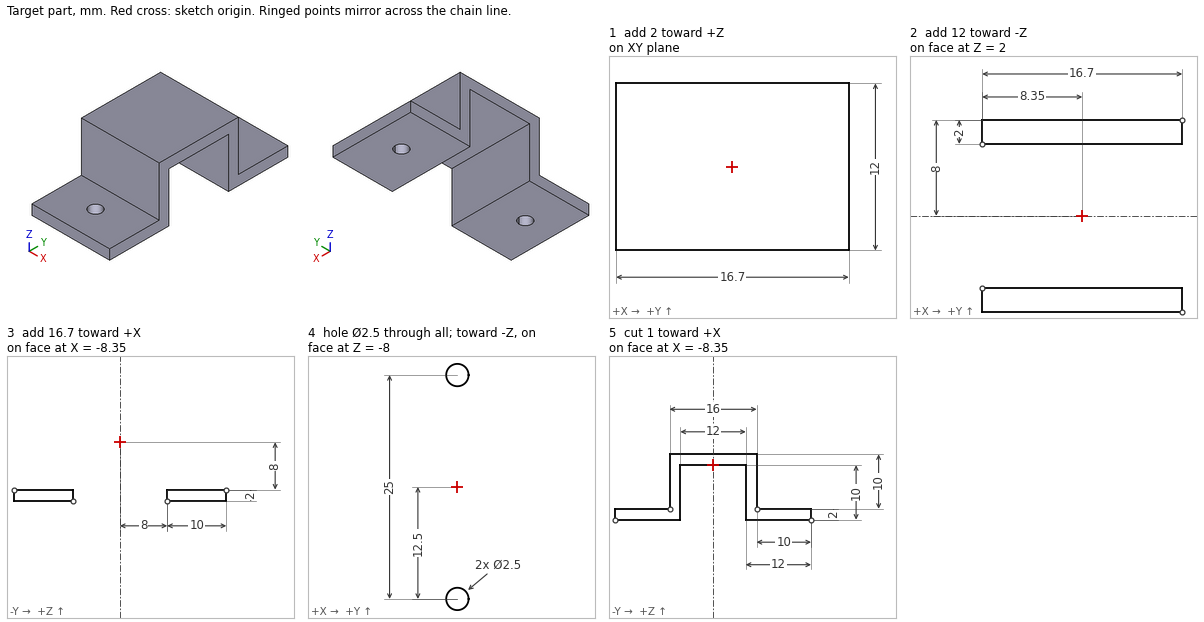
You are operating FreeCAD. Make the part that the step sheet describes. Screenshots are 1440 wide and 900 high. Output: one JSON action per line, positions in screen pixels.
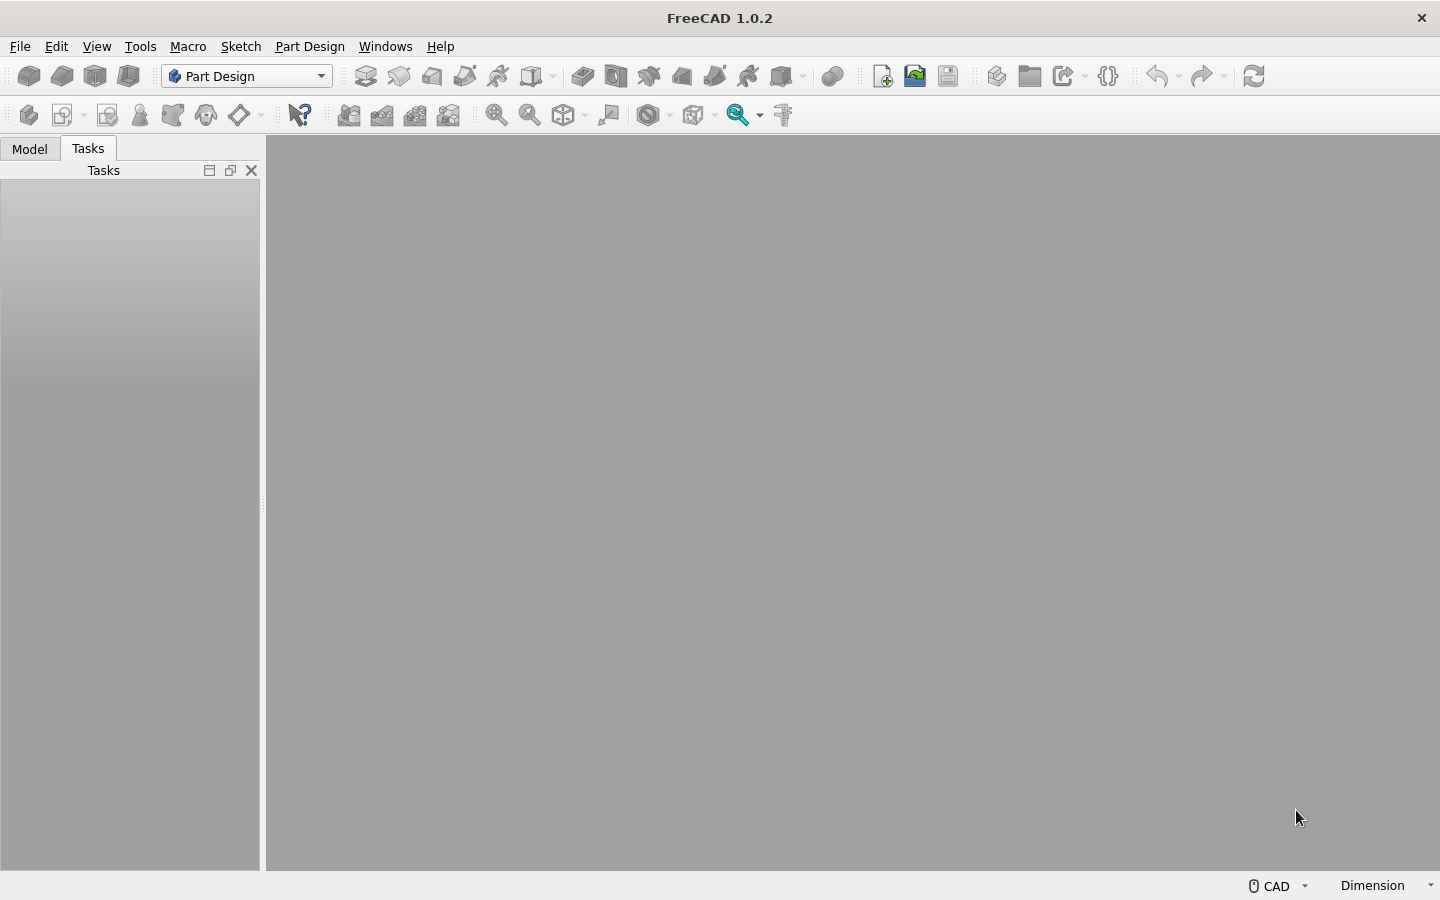
{"action": "left_click", "coordinate": [882, 76]}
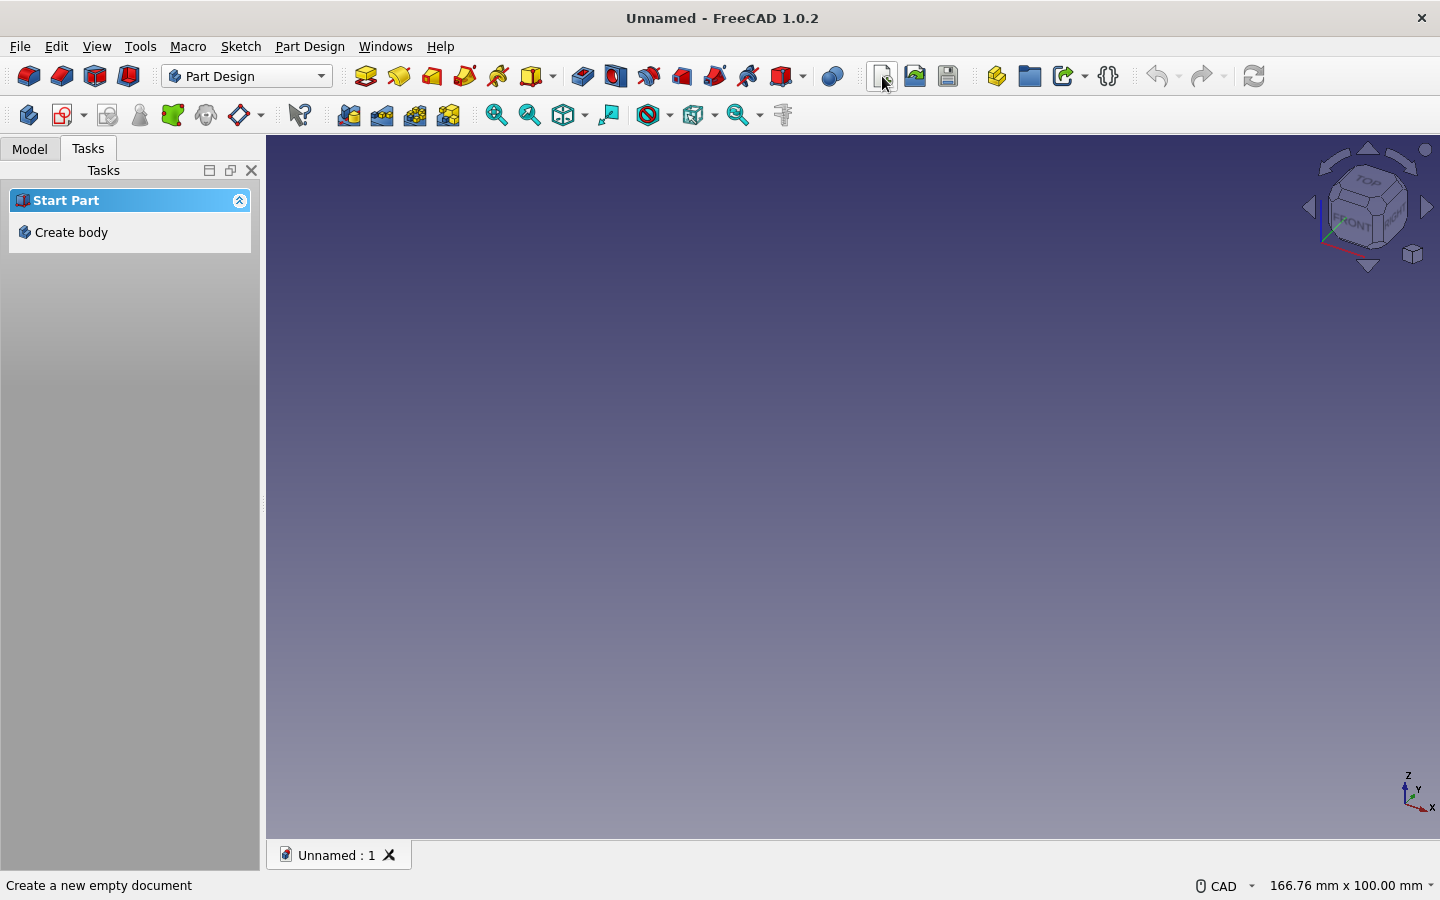
{"action": "left_click", "coordinate": [62, 116]}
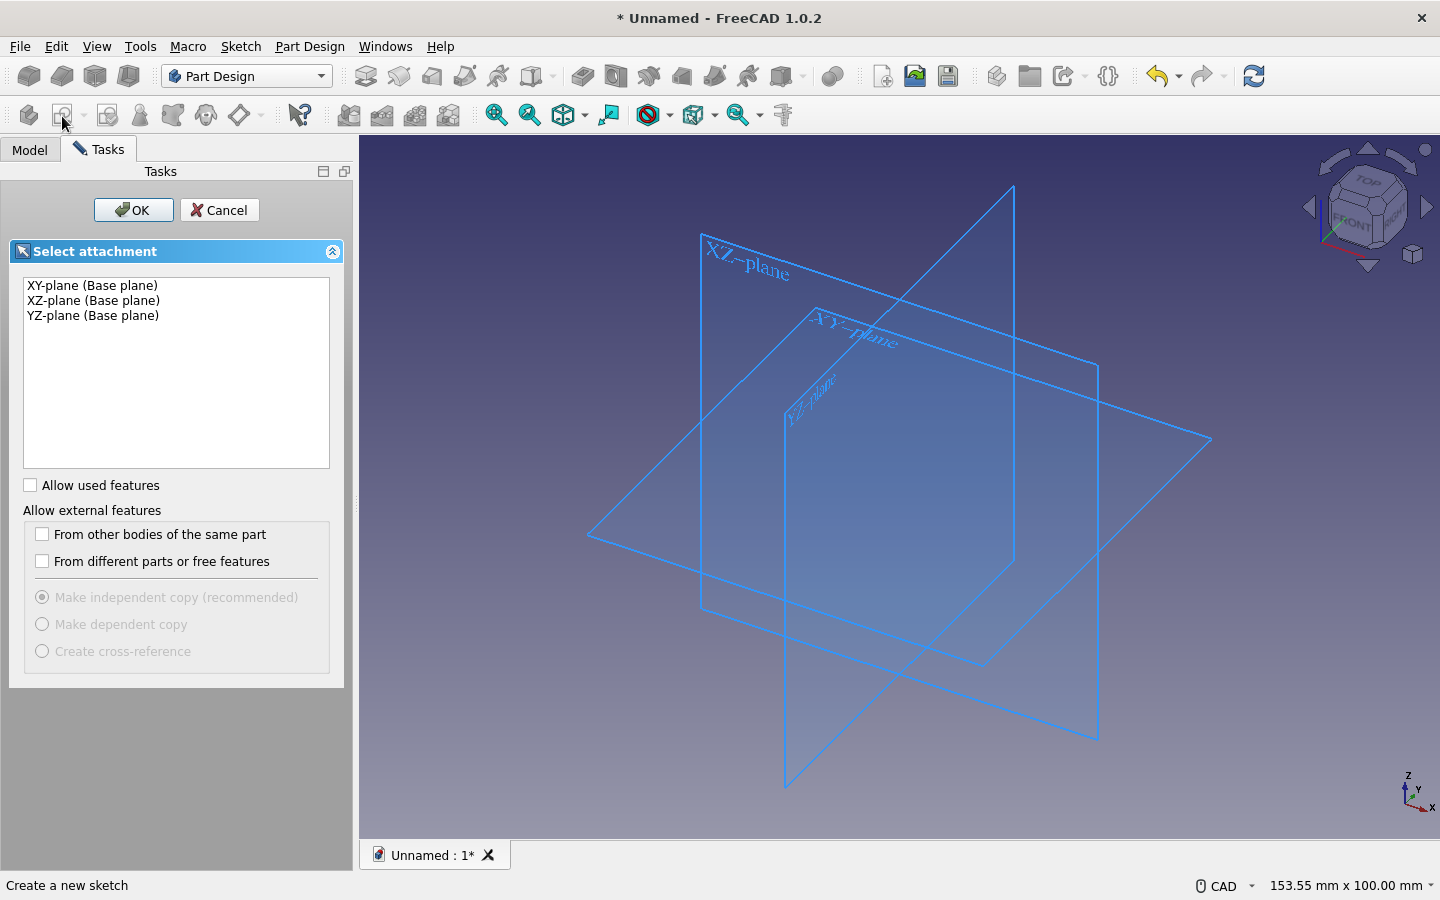
{"action": "left_click", "coordinate": [84, 286]}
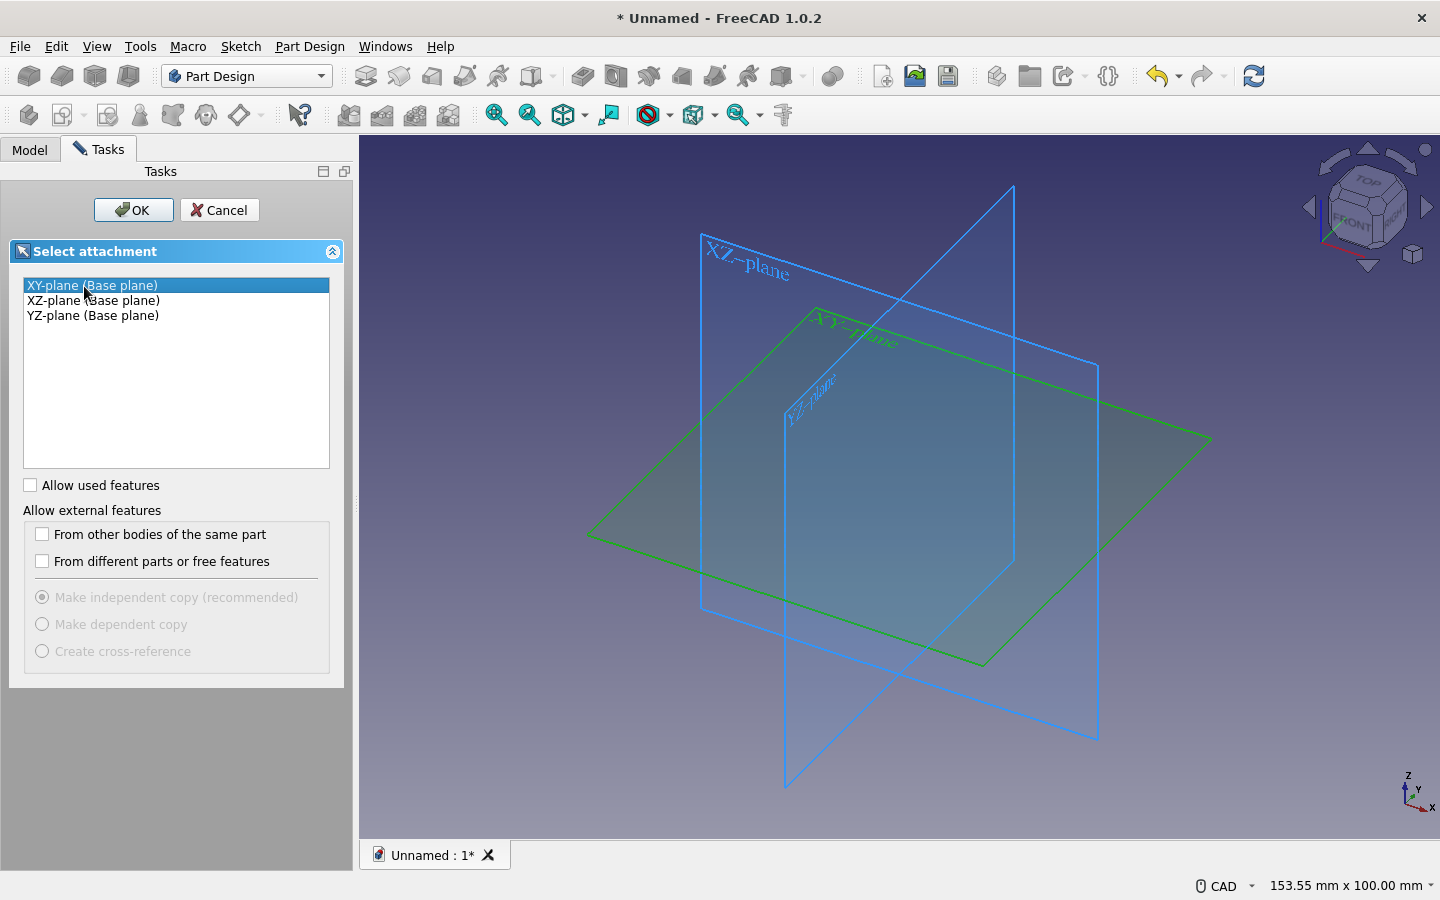
{"action": "left_click", "coordinate": [134, 210]}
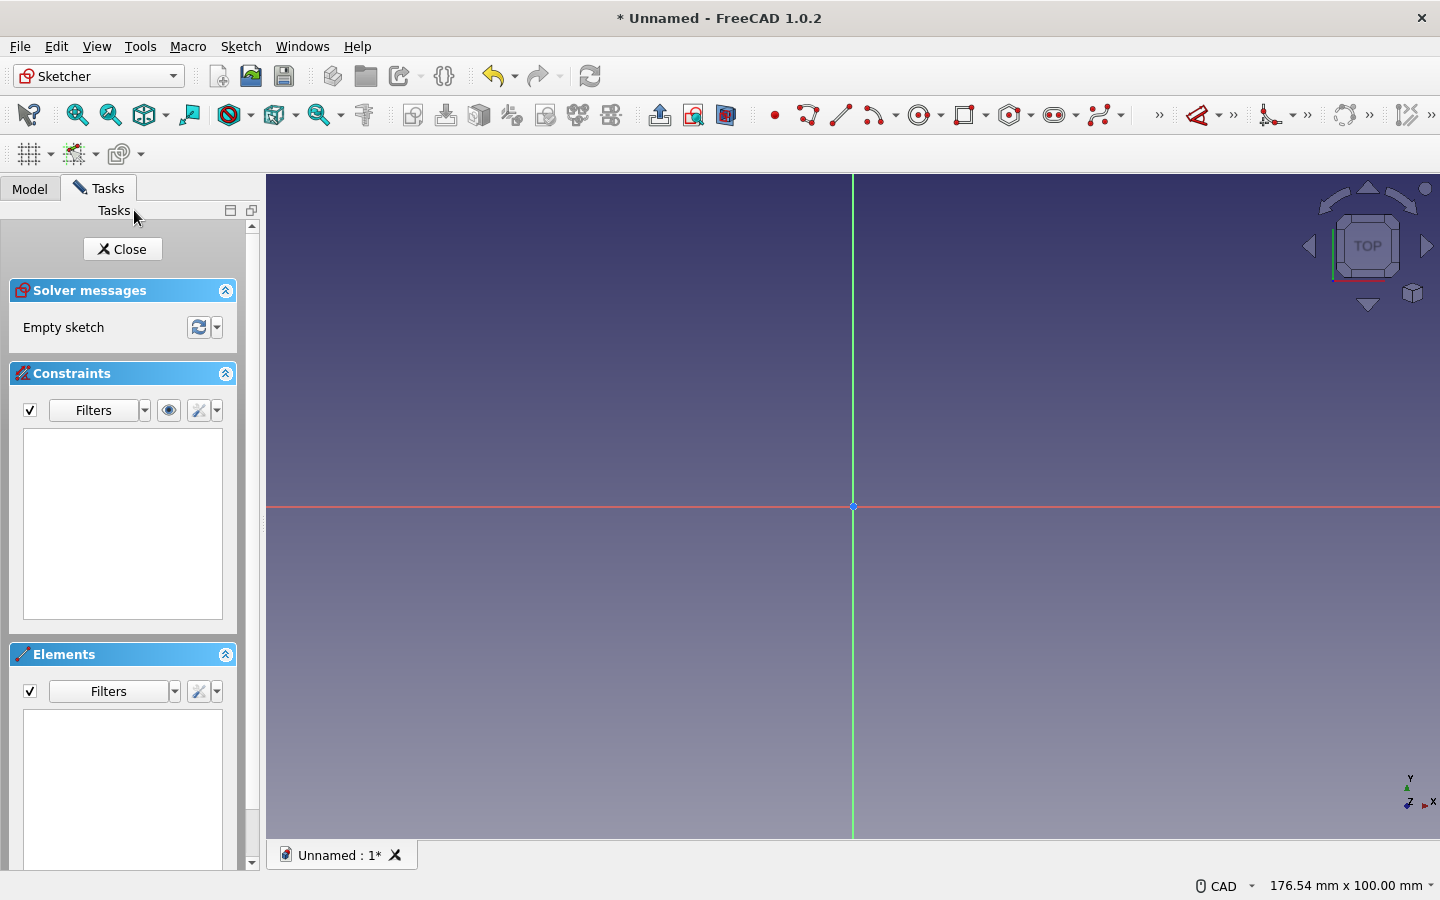
{"action": "scroll", "coordinate": [870, 506], "scroll_direction": "up", "scroll_amount": 8}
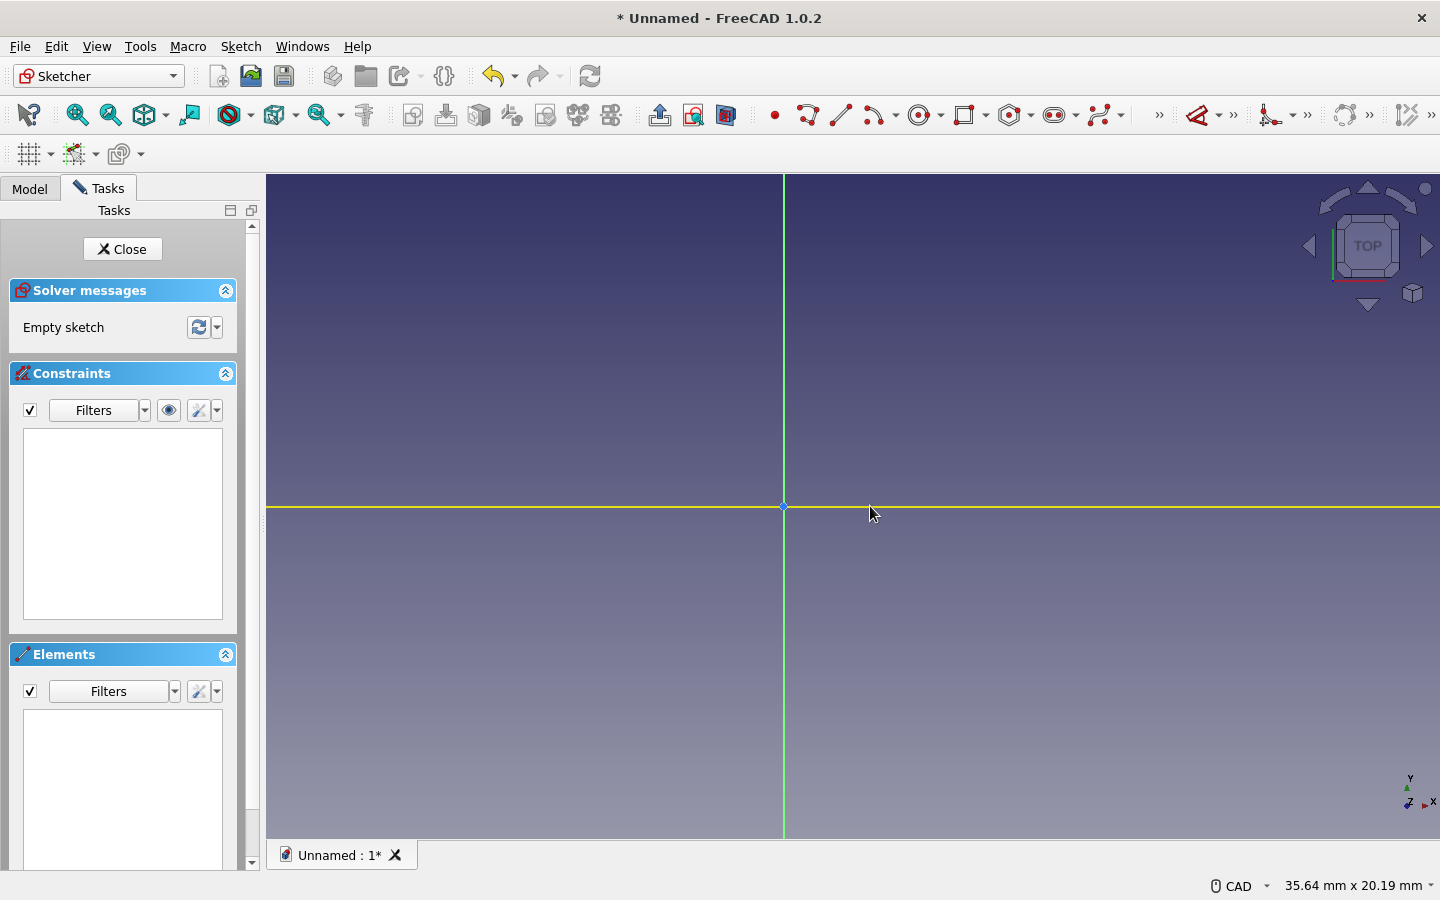
{"action": "left_click", "coordinate": [986, 116]}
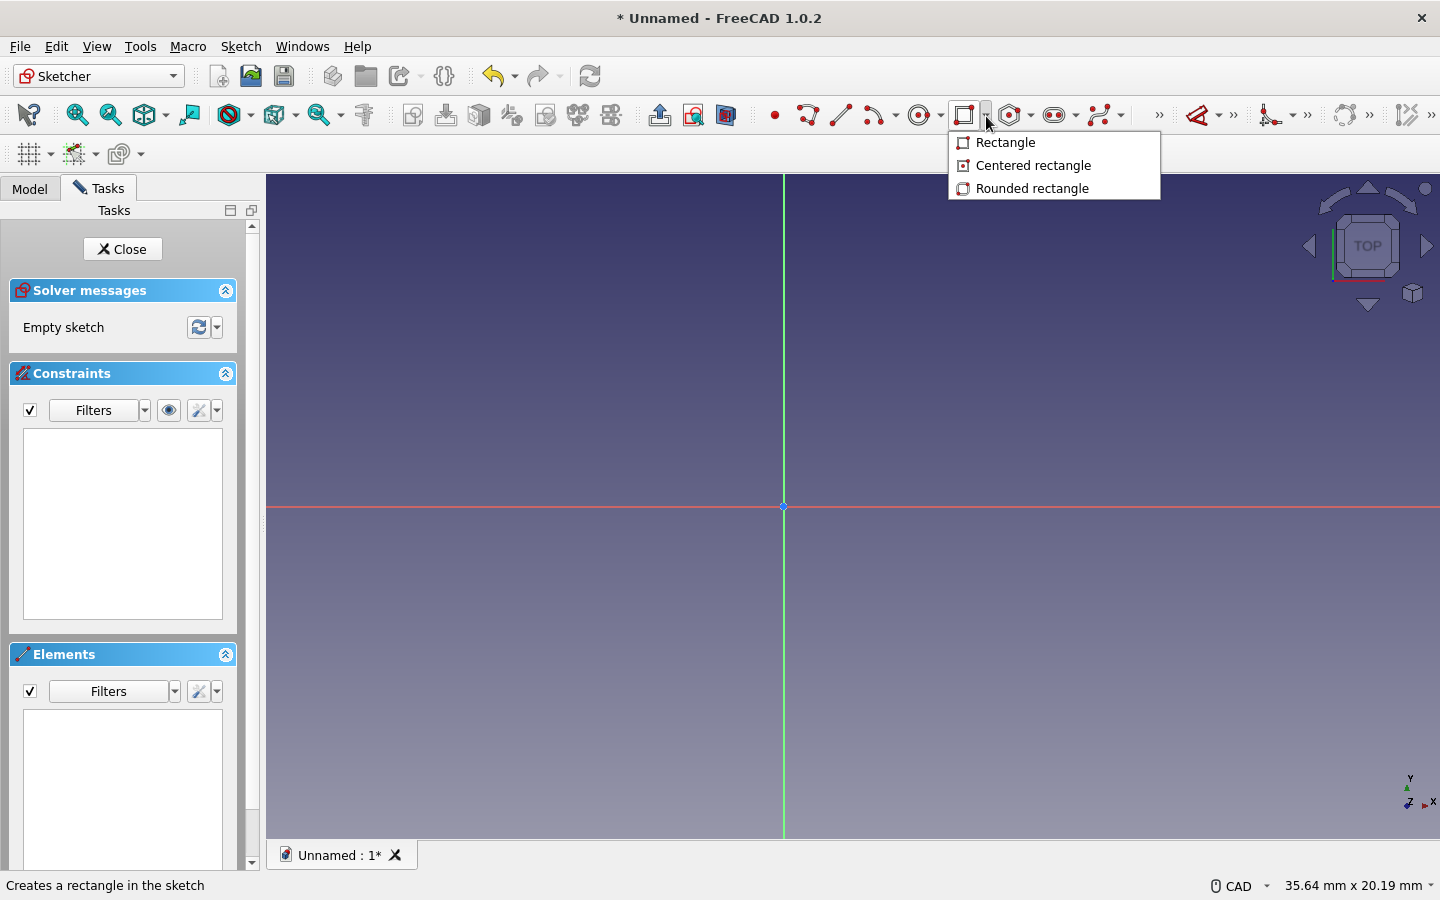
{"action": "left_click", "coordinate": [1054, 166]}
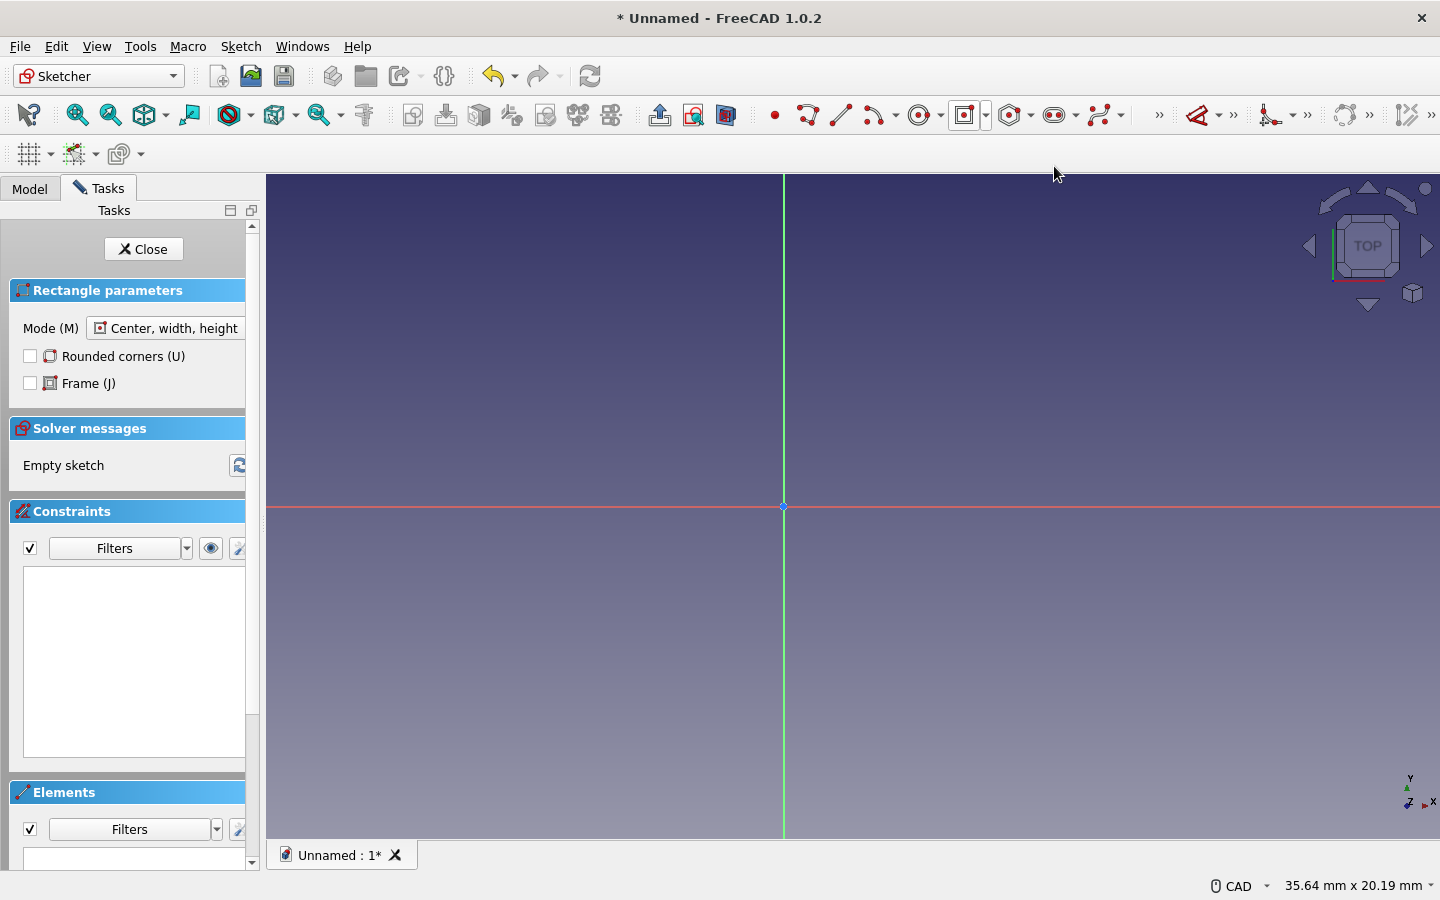
{"action": "left_click", "coordinate": [784, 506]}
{"action": "left_click", "coordinate": [1059, 309]}
{"action": "key", "text": "Escape"}